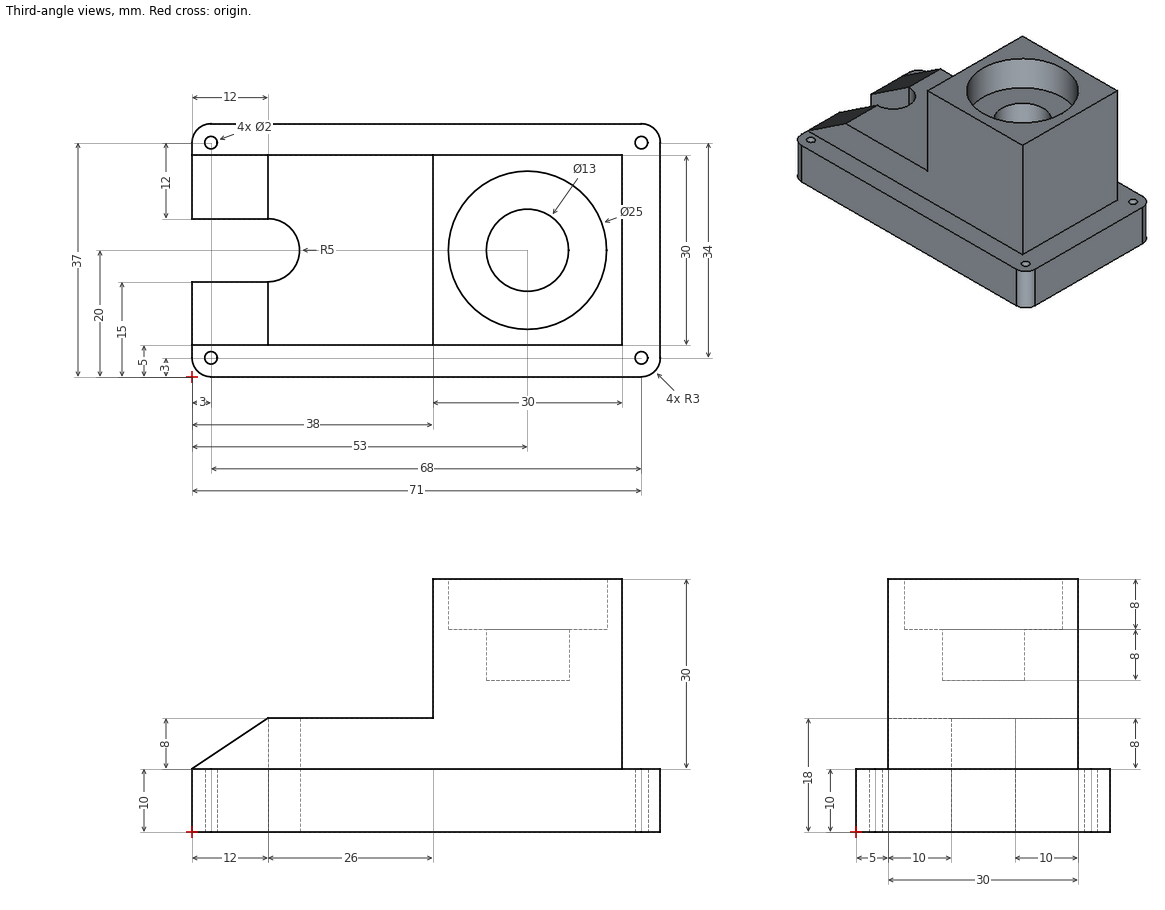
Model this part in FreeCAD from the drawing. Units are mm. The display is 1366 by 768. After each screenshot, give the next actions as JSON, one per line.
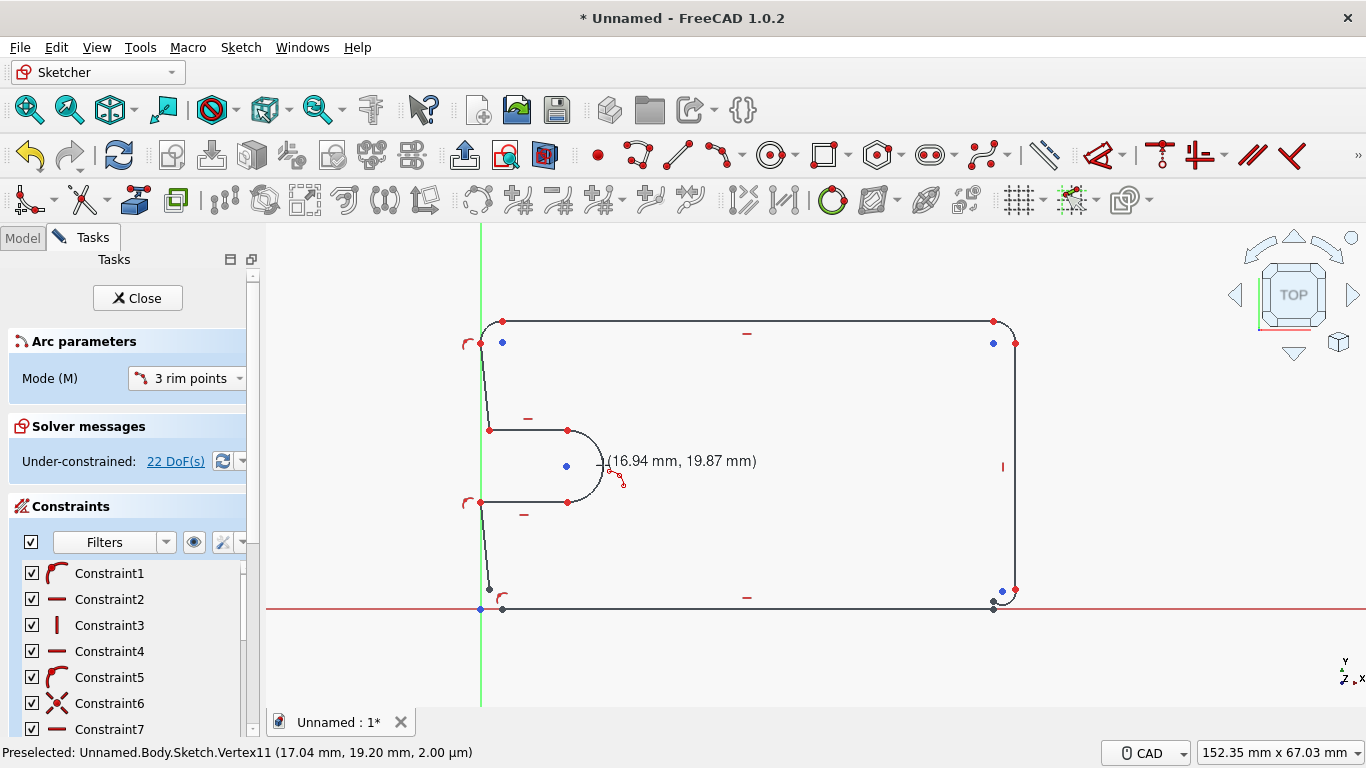
{"action": "left_click", "coordinate": [489, 589]}
{"action": "left_click", "coordinate": [502, 609]}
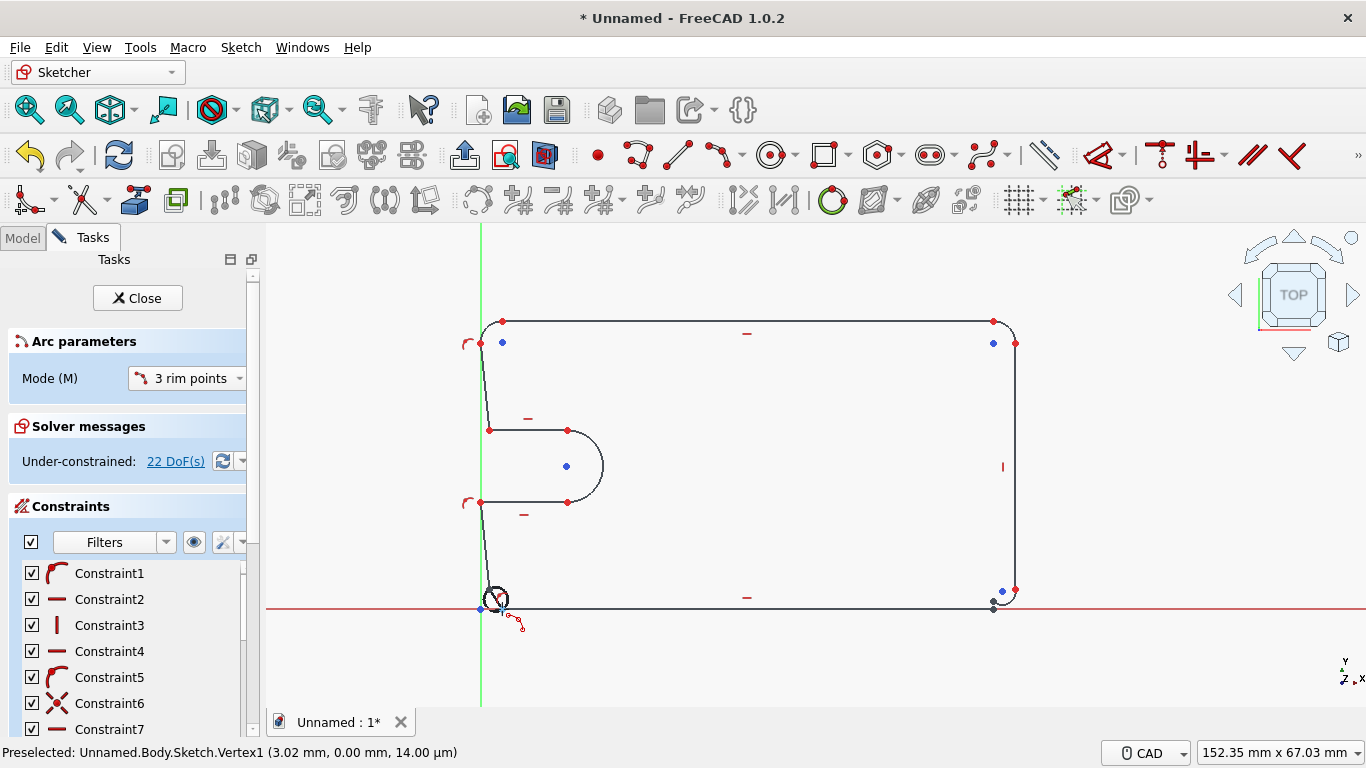
{"action": "scroll", "coordinate": [487, 603], "scroll_direction": "up", "scroll_amount": 5}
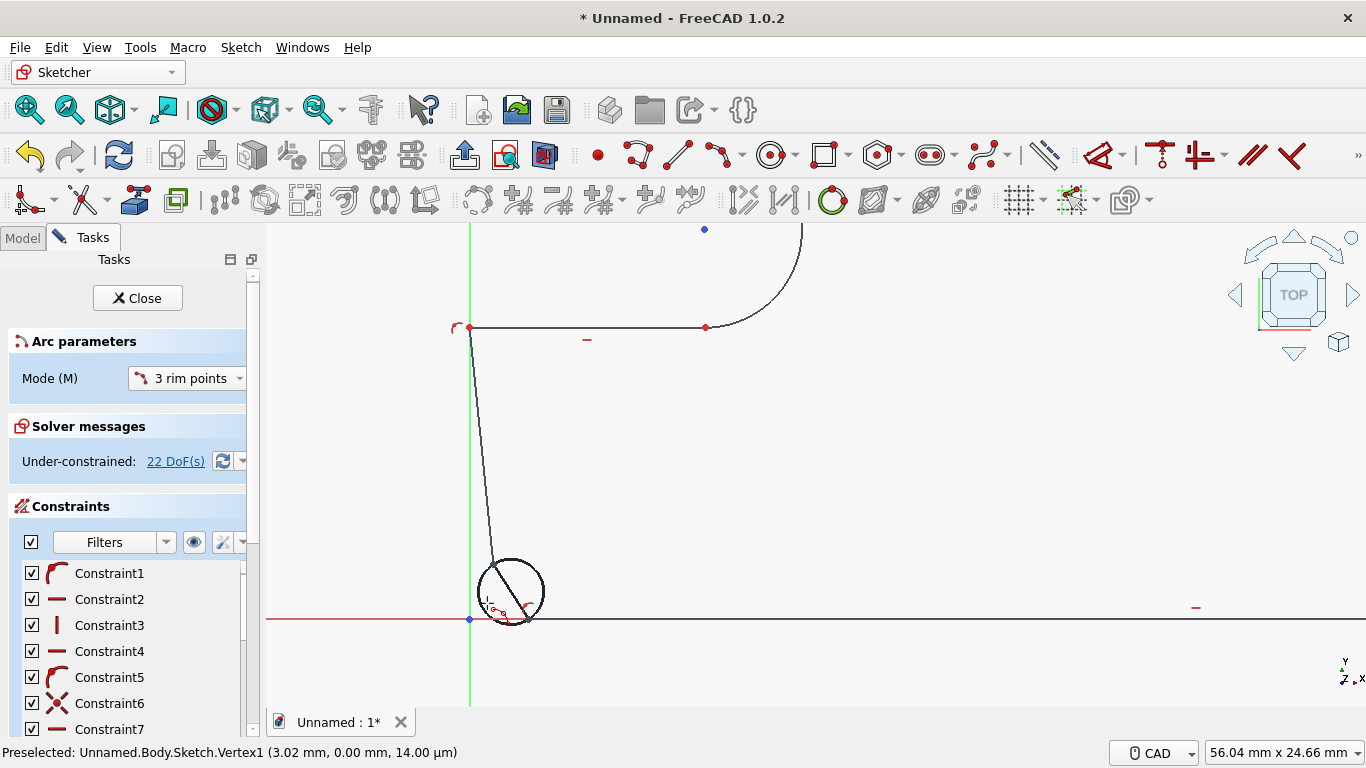
{"action": "left_click", "coordinate": [487, 602]}
{"action": "key", "text": "Escape"}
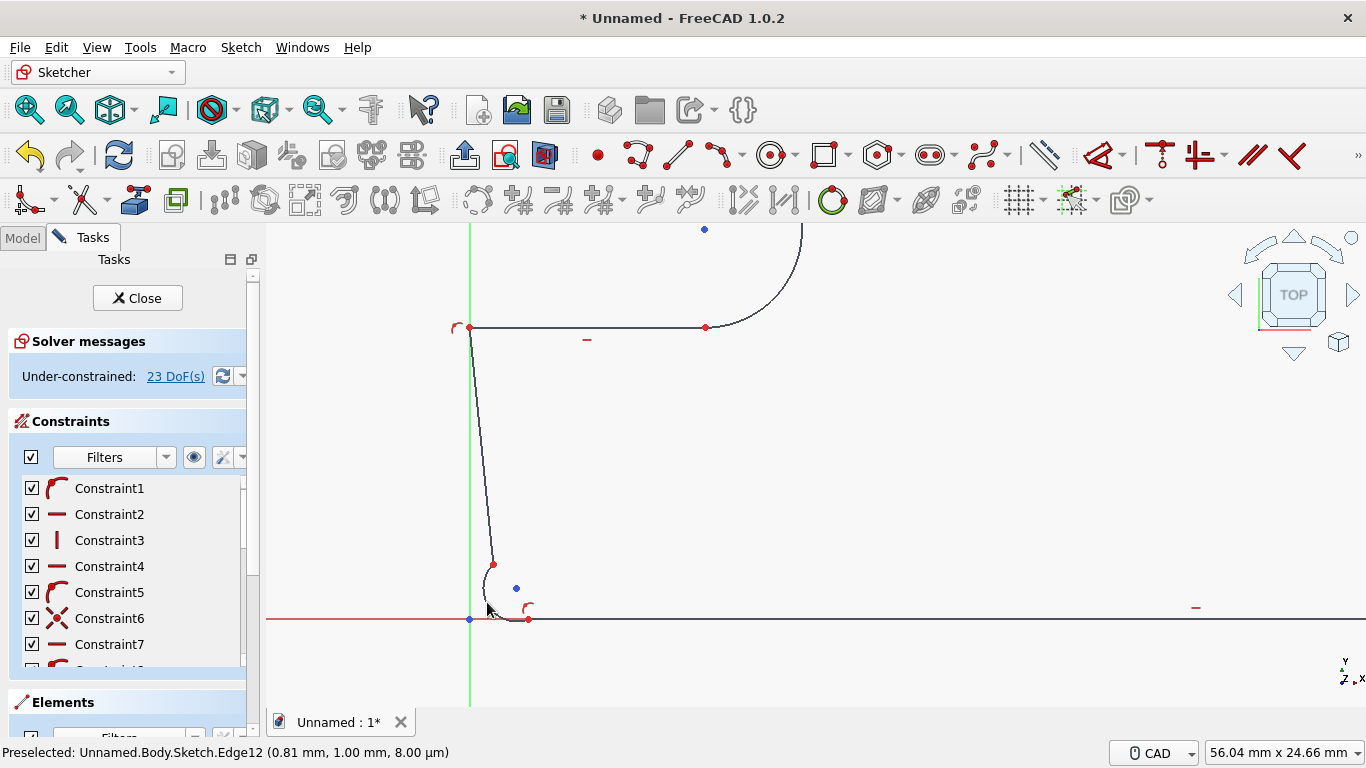
{"action": "left_click", "coordinate": [929, 619]}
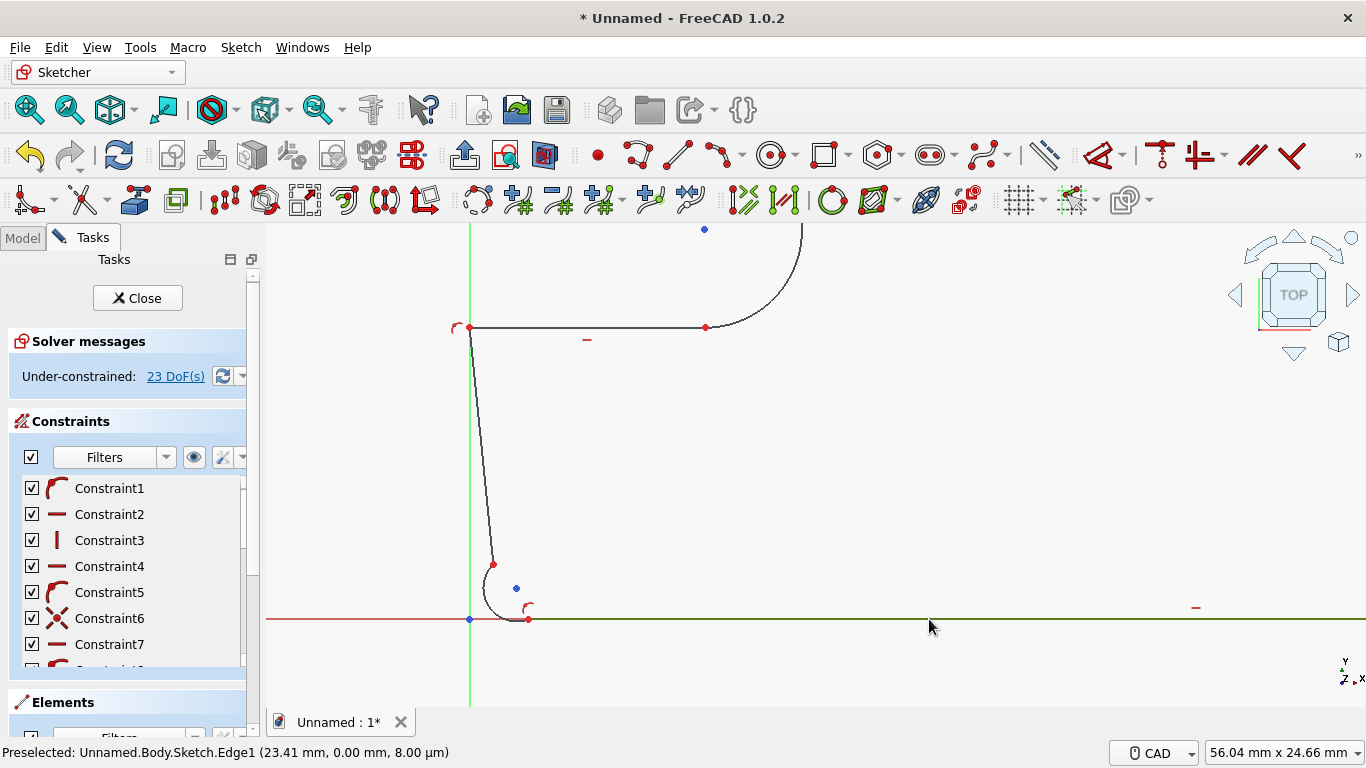
{"action": "scroll", "coordinate": [487, 604], "scroll_direction": "down", "scroll_amount": 5}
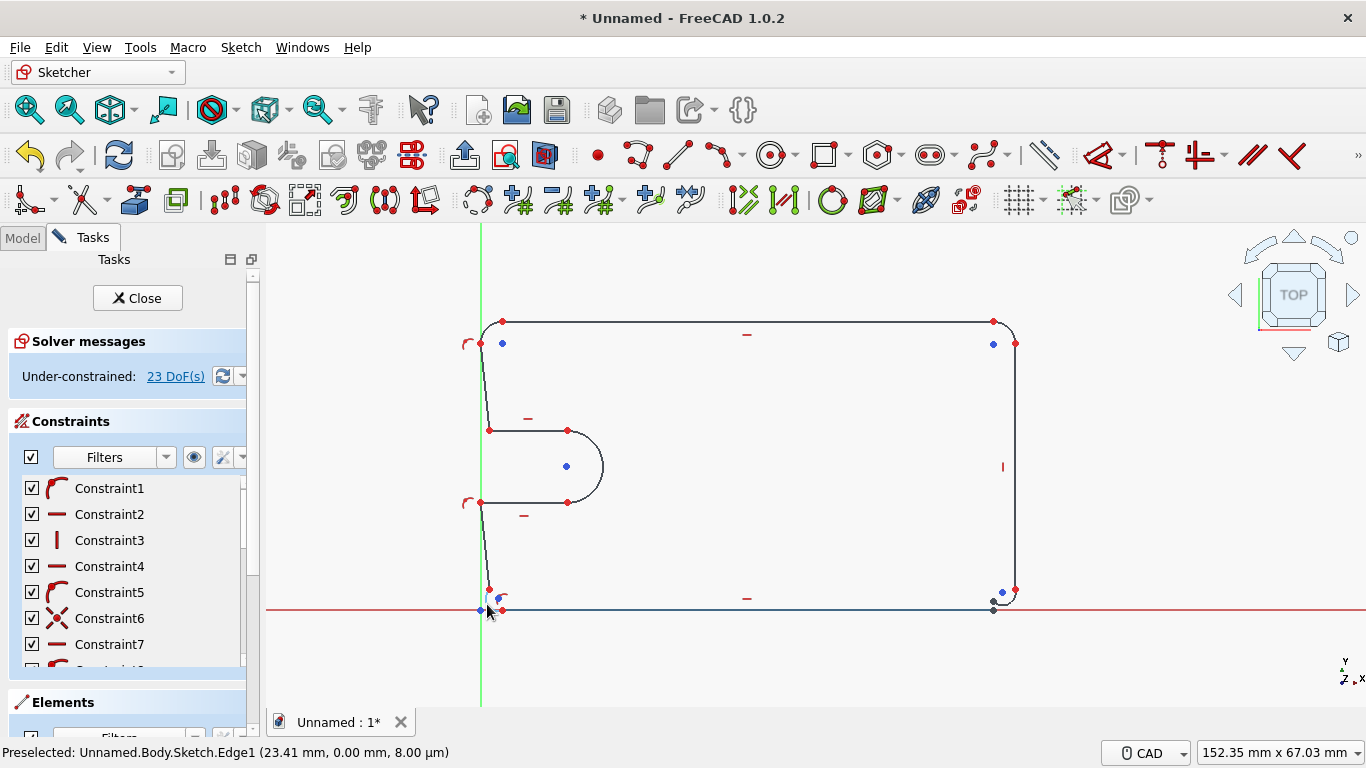
{"action": "scroll", "coordinate": [1002, 605], "scroll_direction": "up", "scroll_amount": 6}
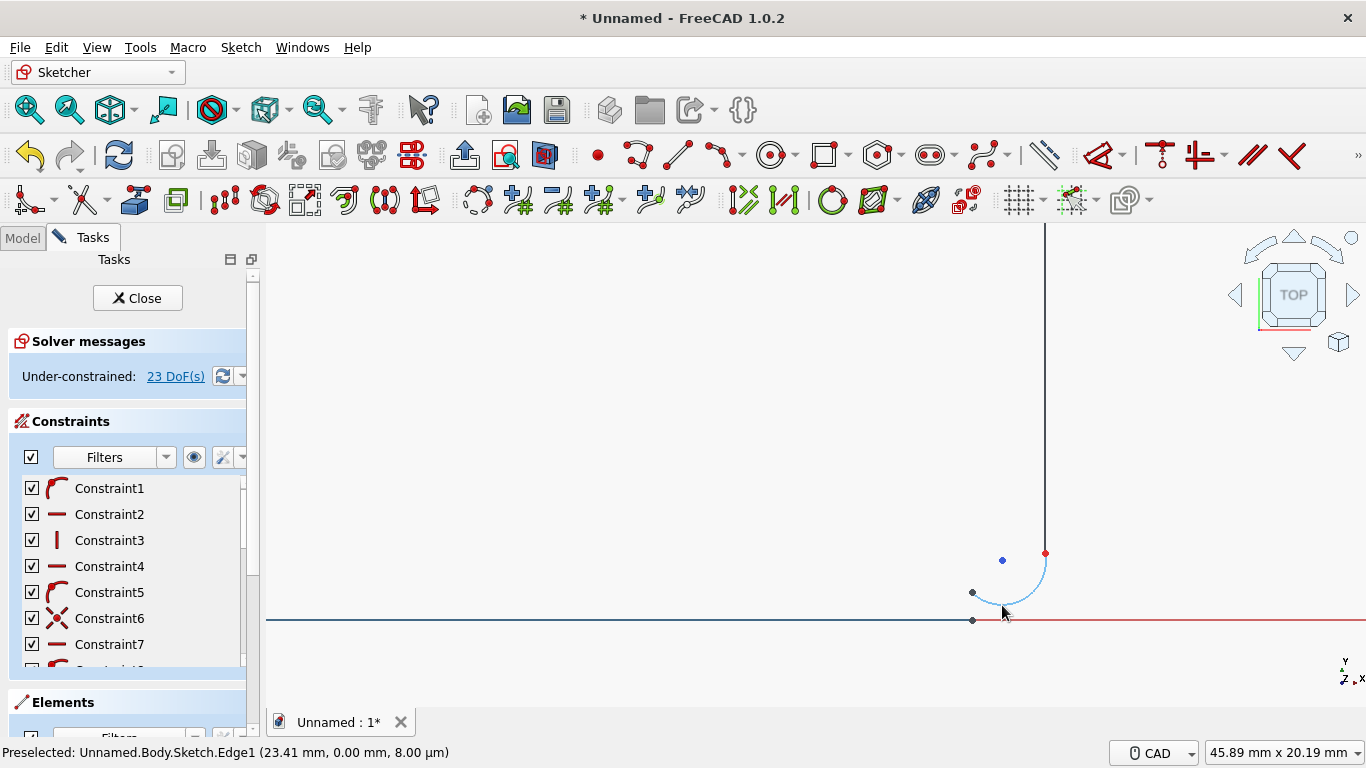
{"action": "left_click", "coordinate": [1002, 605]}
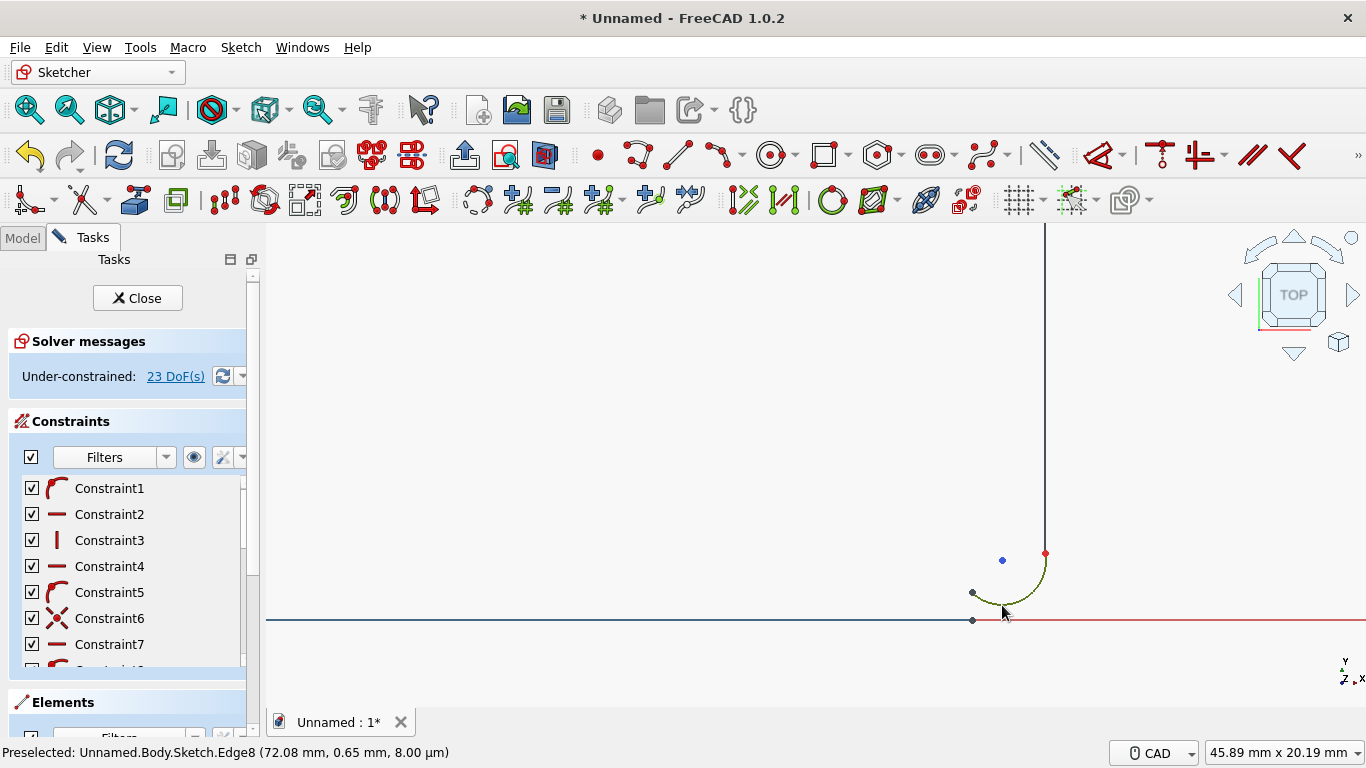
{"action": "key", "text": "t"}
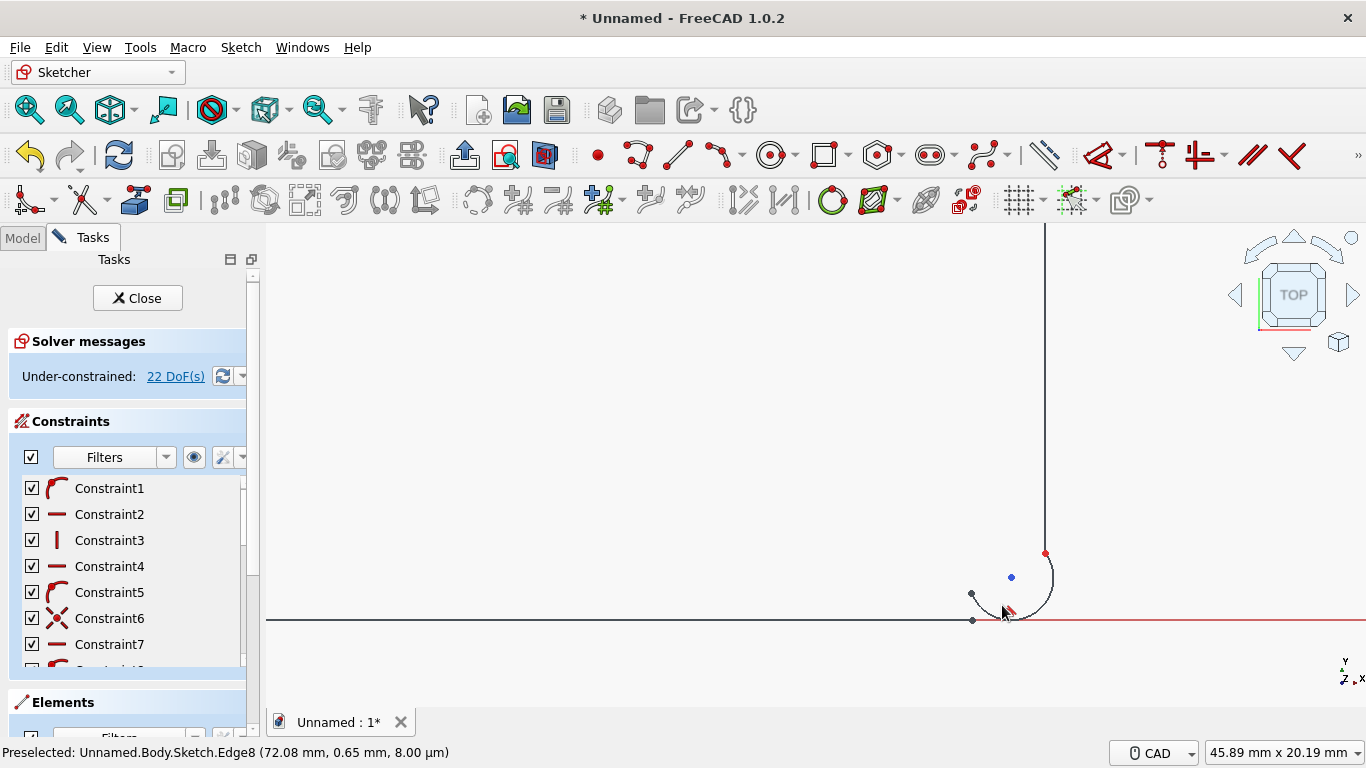
{"action": "left_click", "coordinate": [483, 620]}